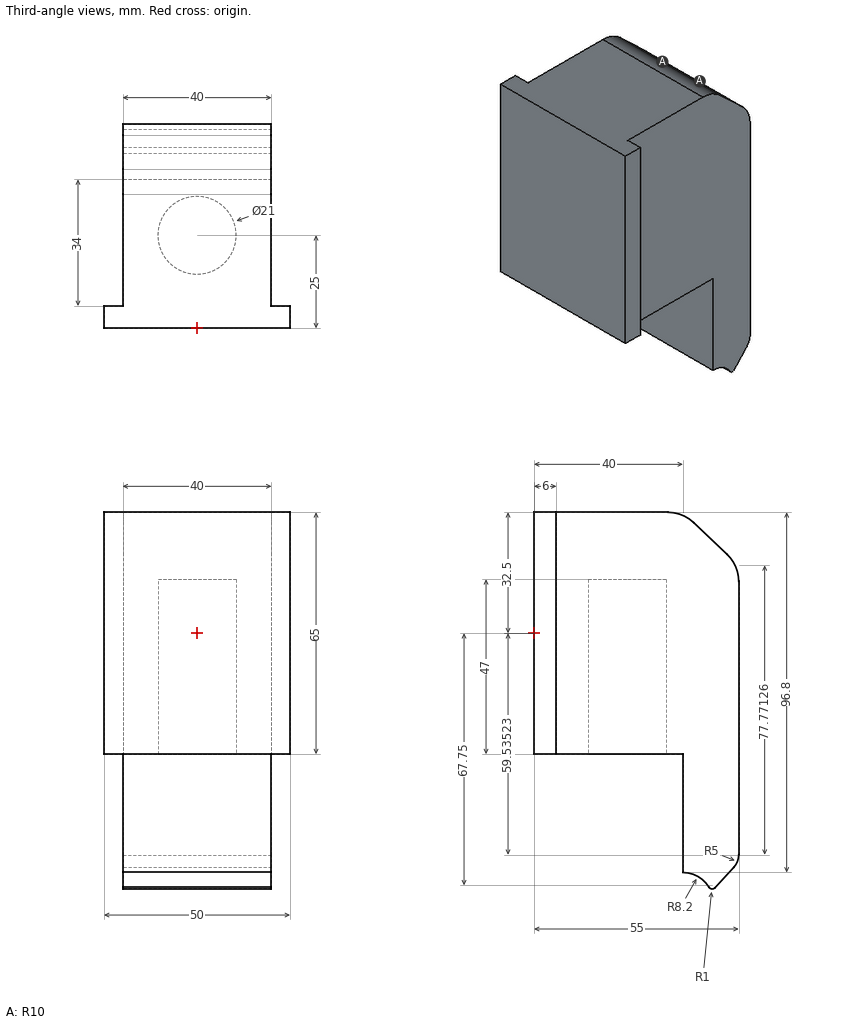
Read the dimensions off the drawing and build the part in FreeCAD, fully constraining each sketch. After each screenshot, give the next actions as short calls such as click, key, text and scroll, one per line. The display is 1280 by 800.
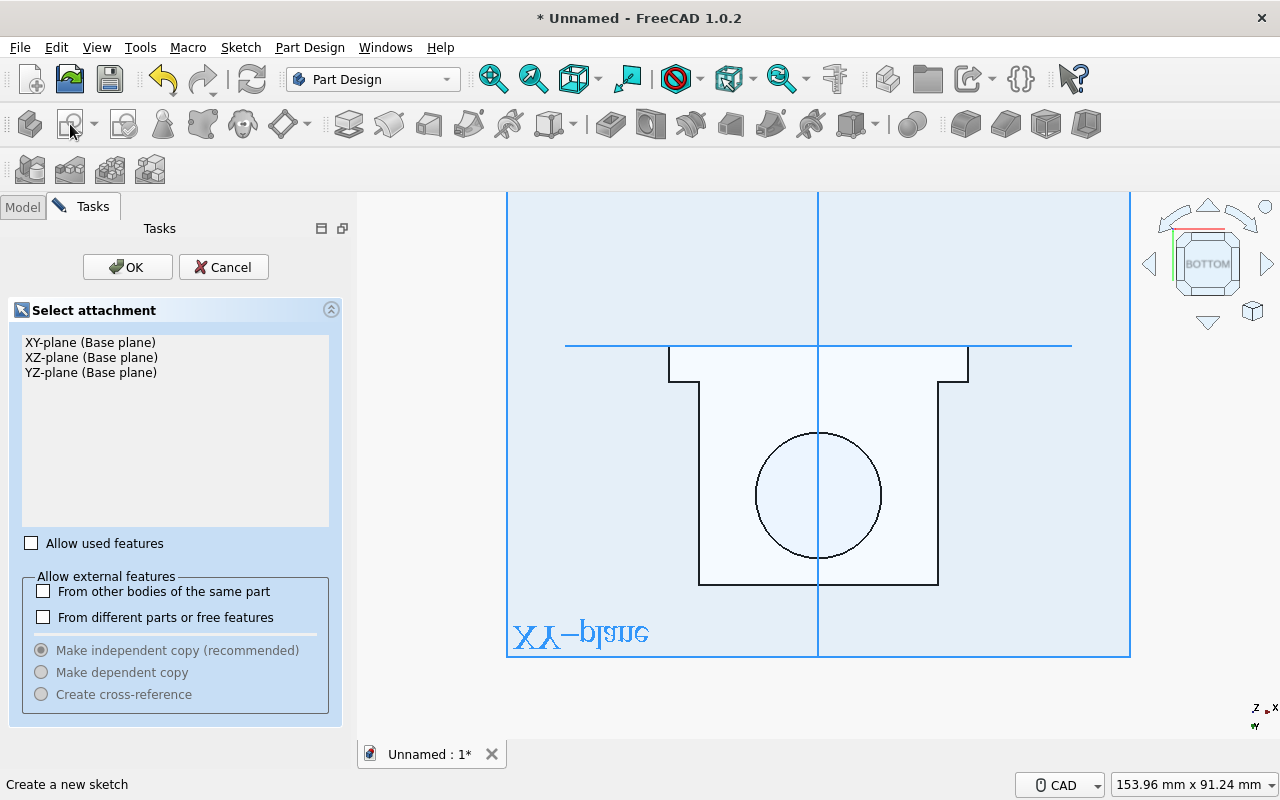
click(82, 372)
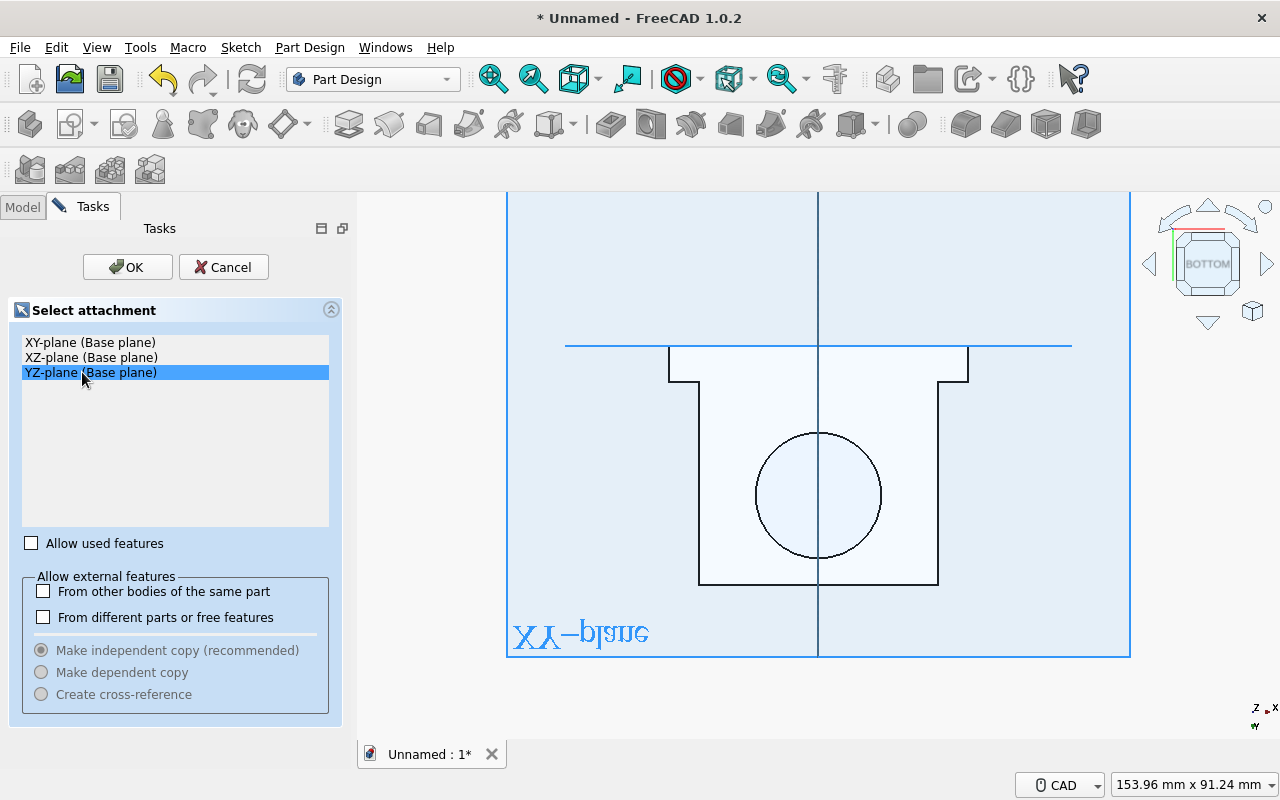
click(128, 267)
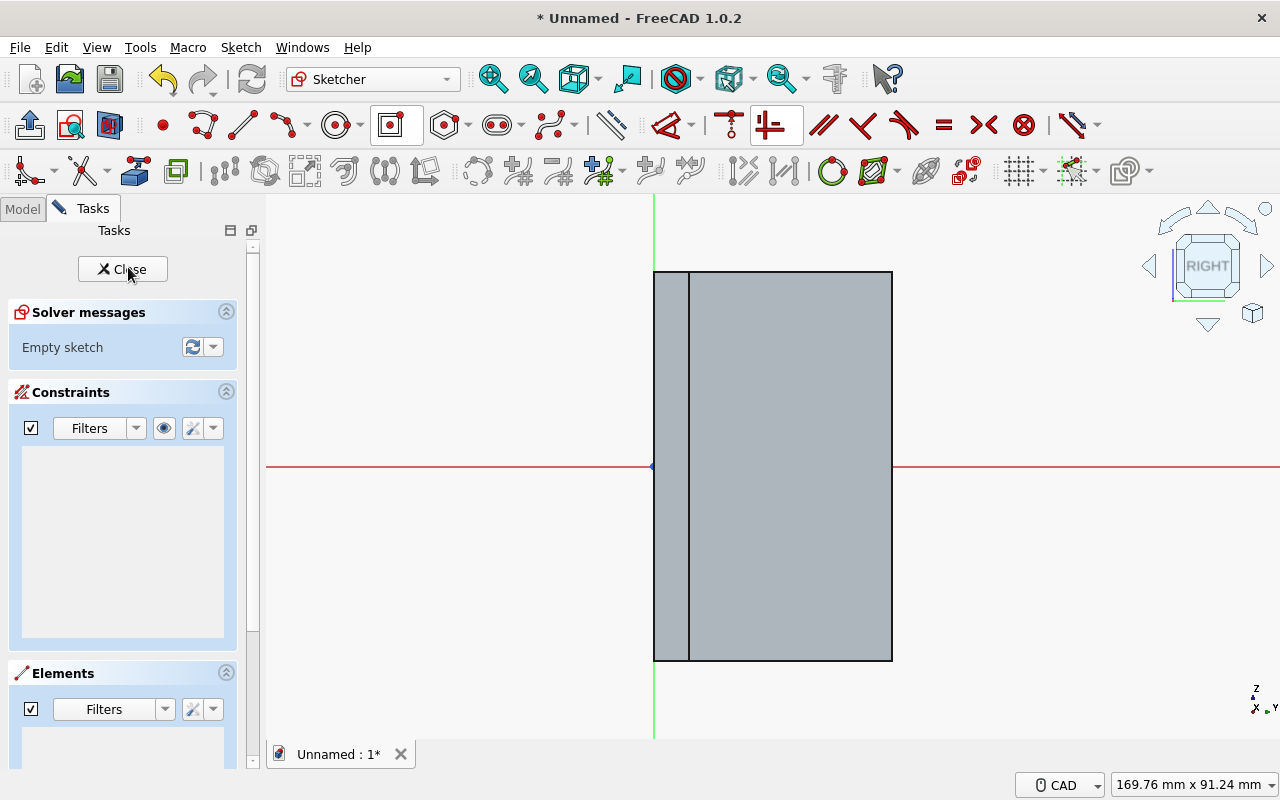
click(110, 126)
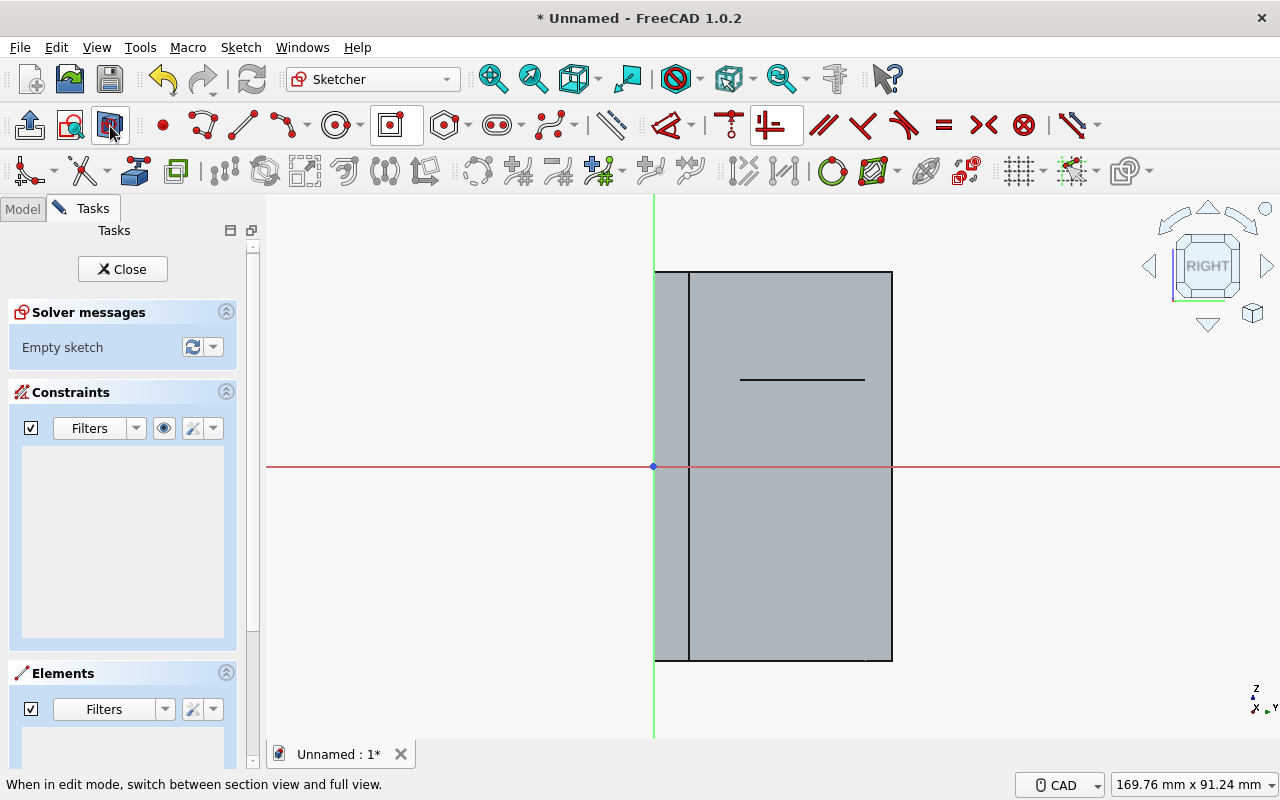
scroll(567, 335, down, 3)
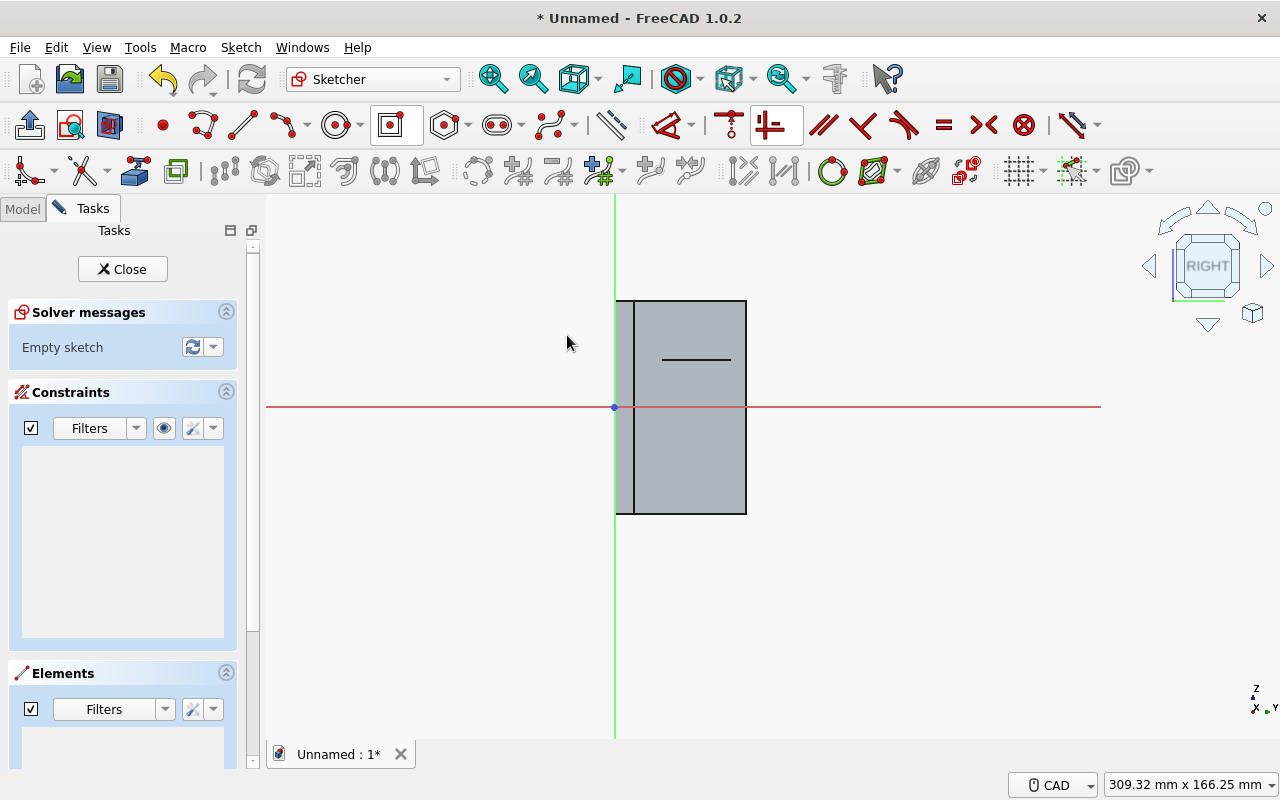
click(244, 126)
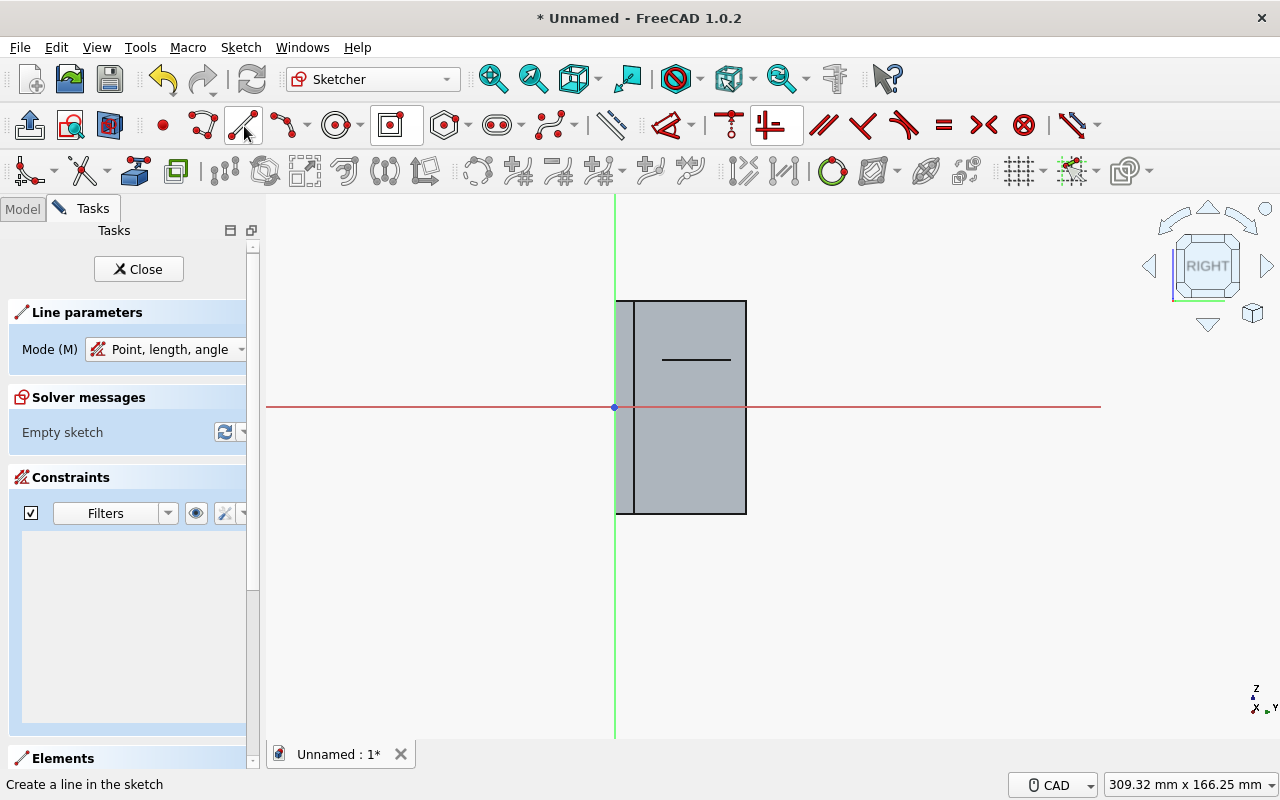
click(774, 632)
click(791, 614)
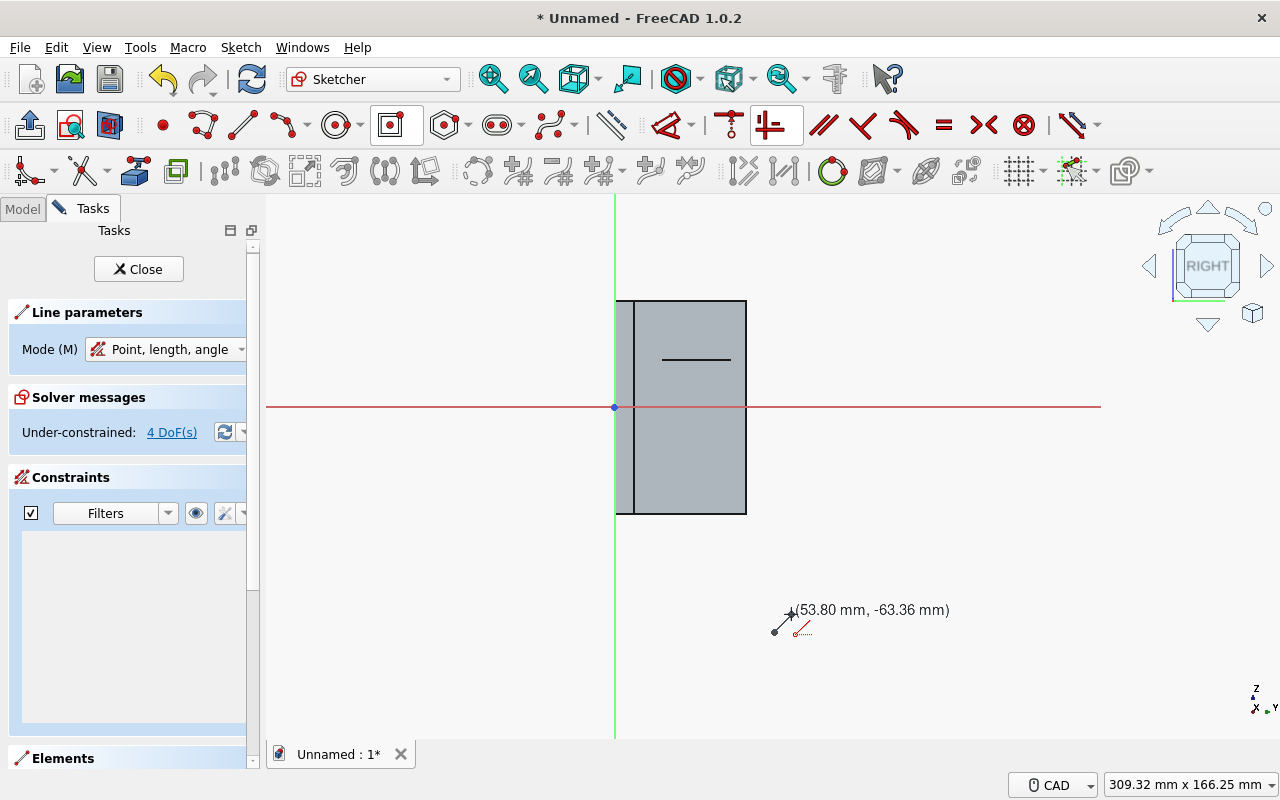
click(204, 126)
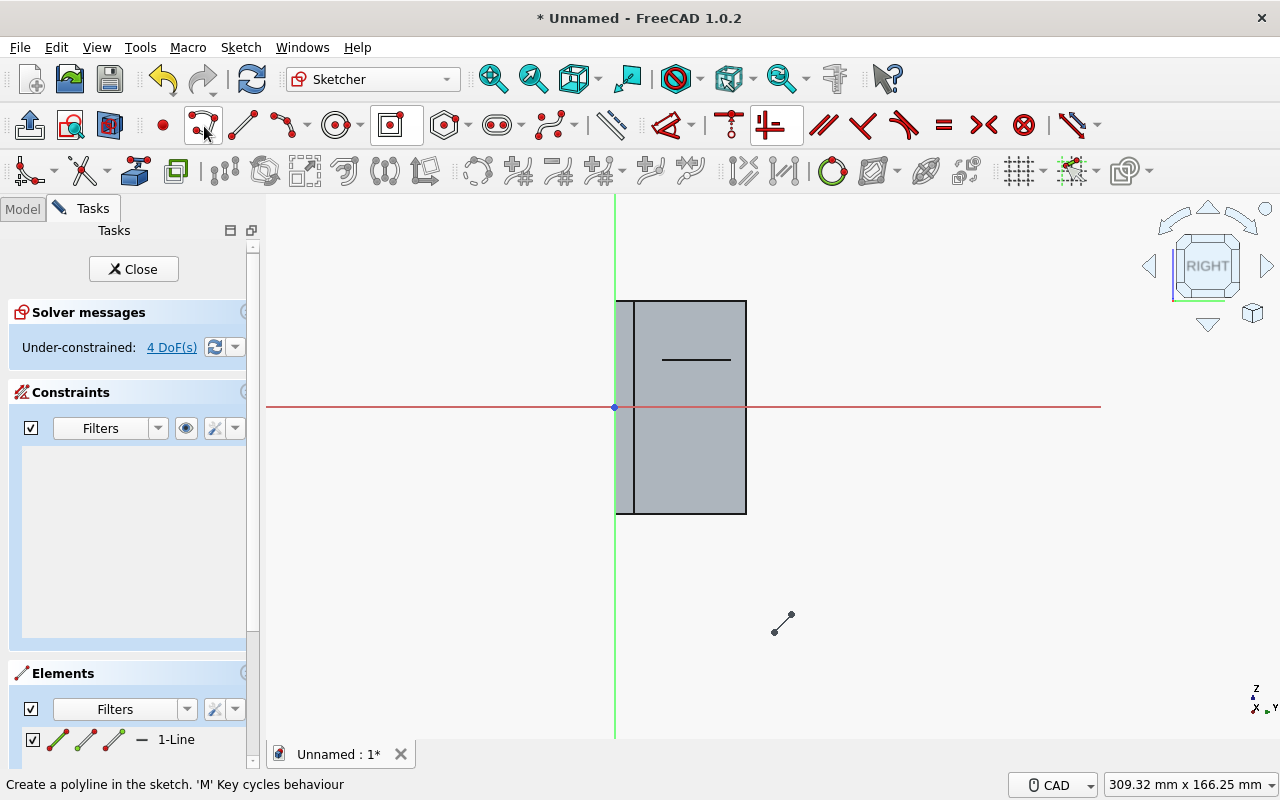
scroll(795, 602, up, 2)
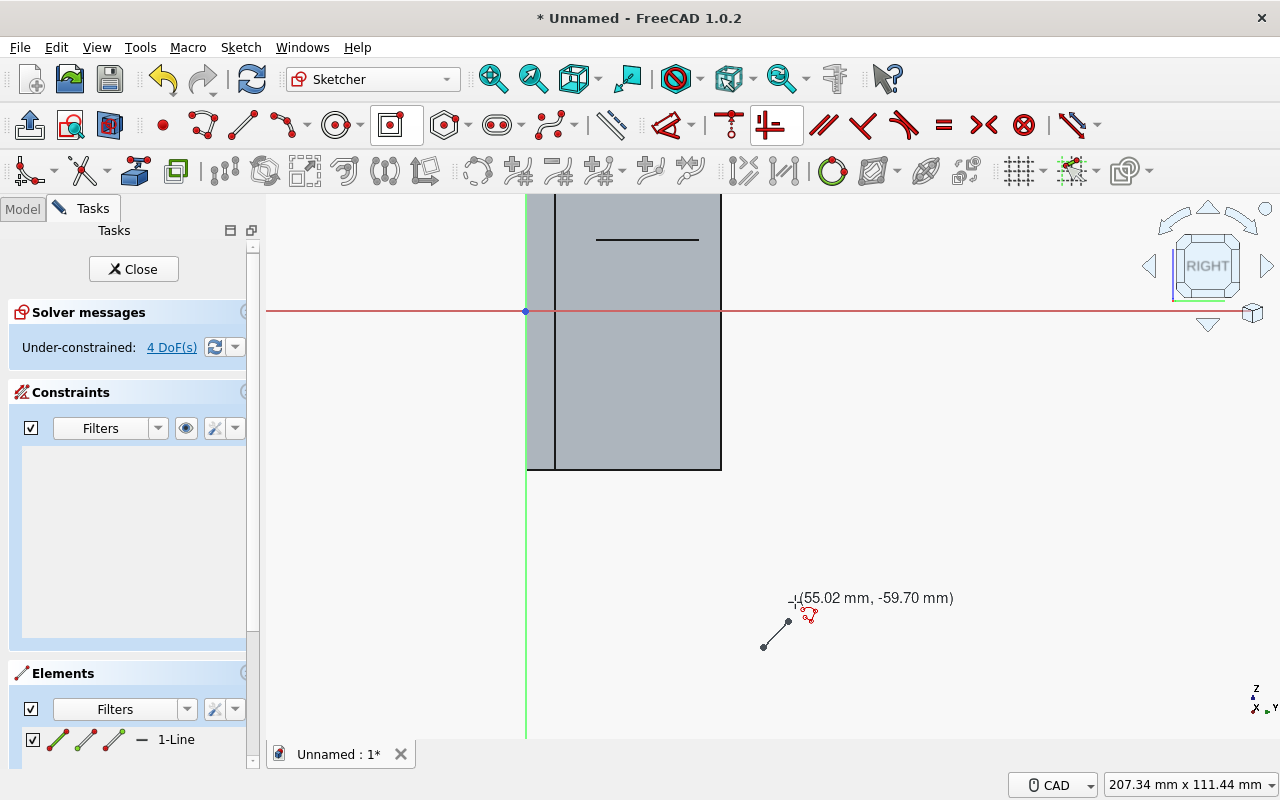
click(795, 602)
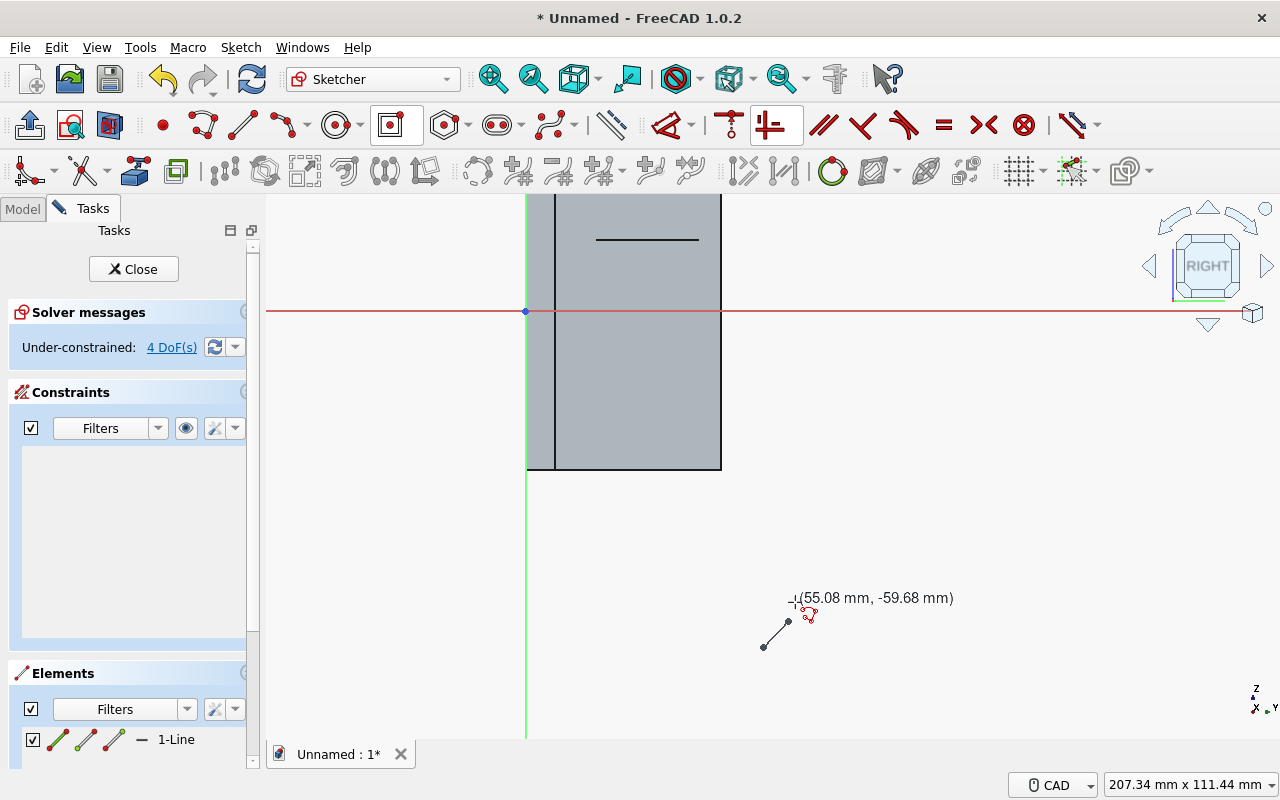
scroll(795, 602, down, 2)